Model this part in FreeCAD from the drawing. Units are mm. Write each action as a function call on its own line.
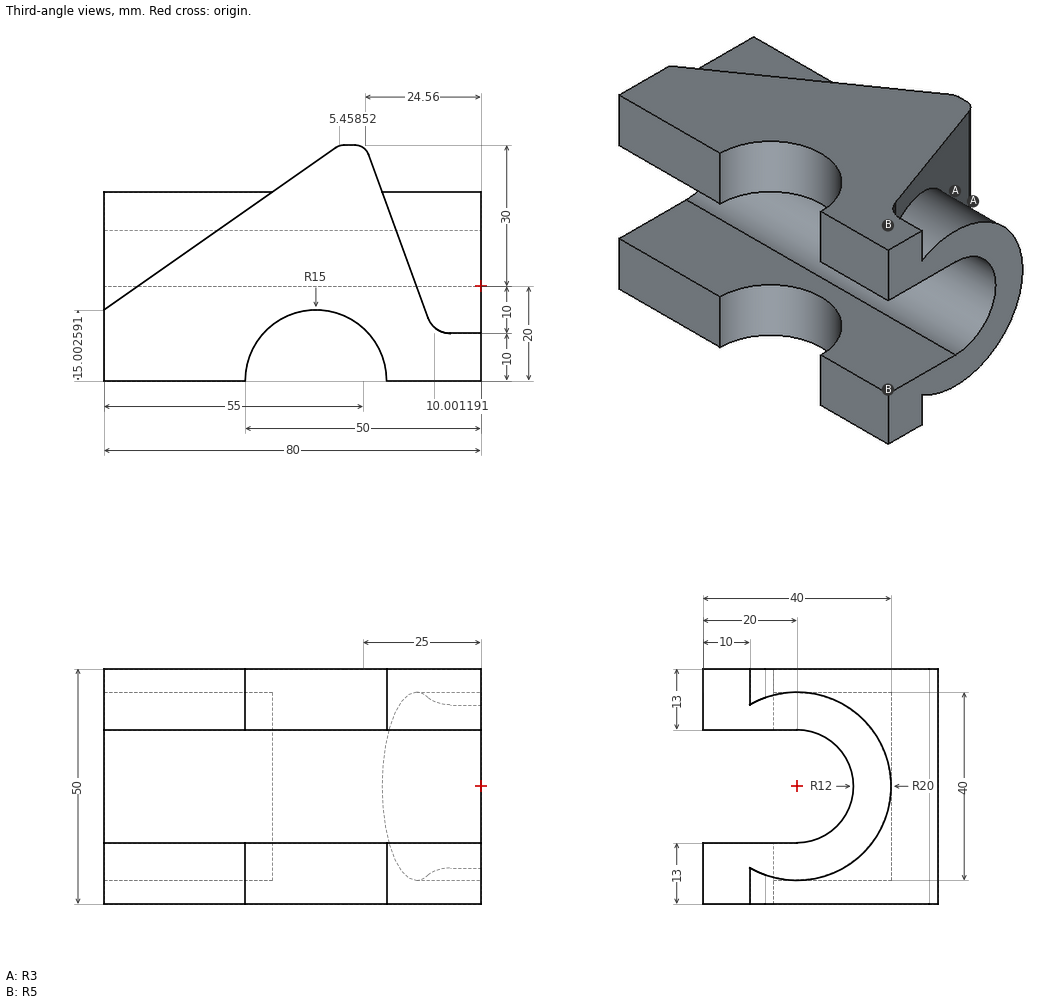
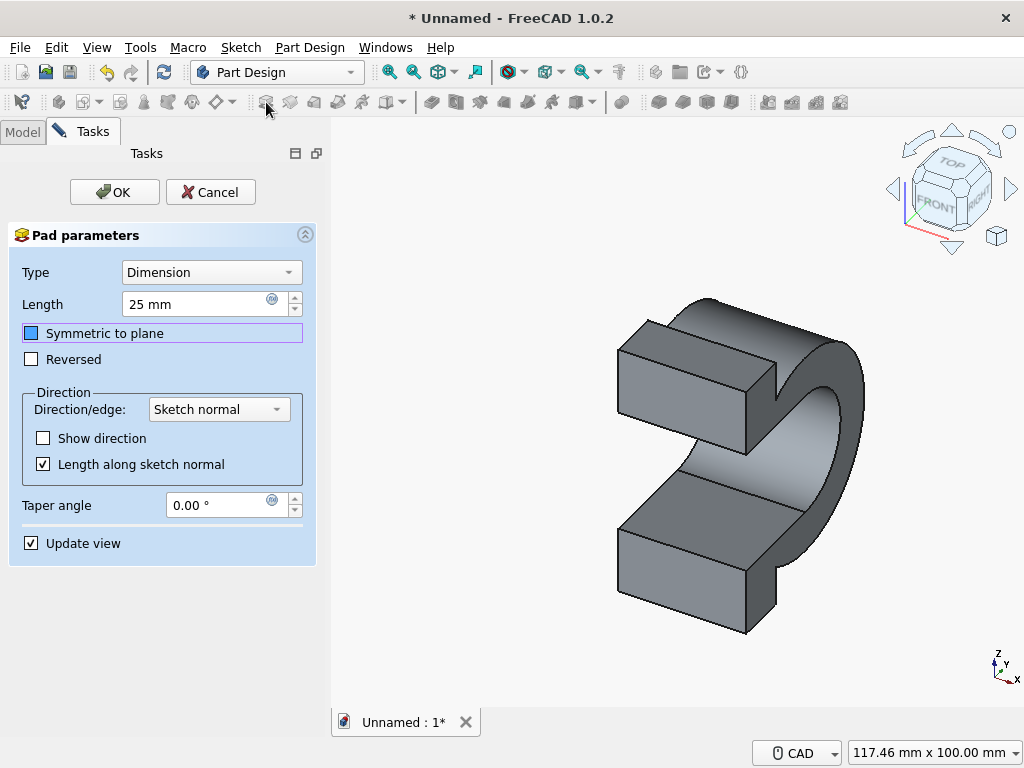
click(30, 359)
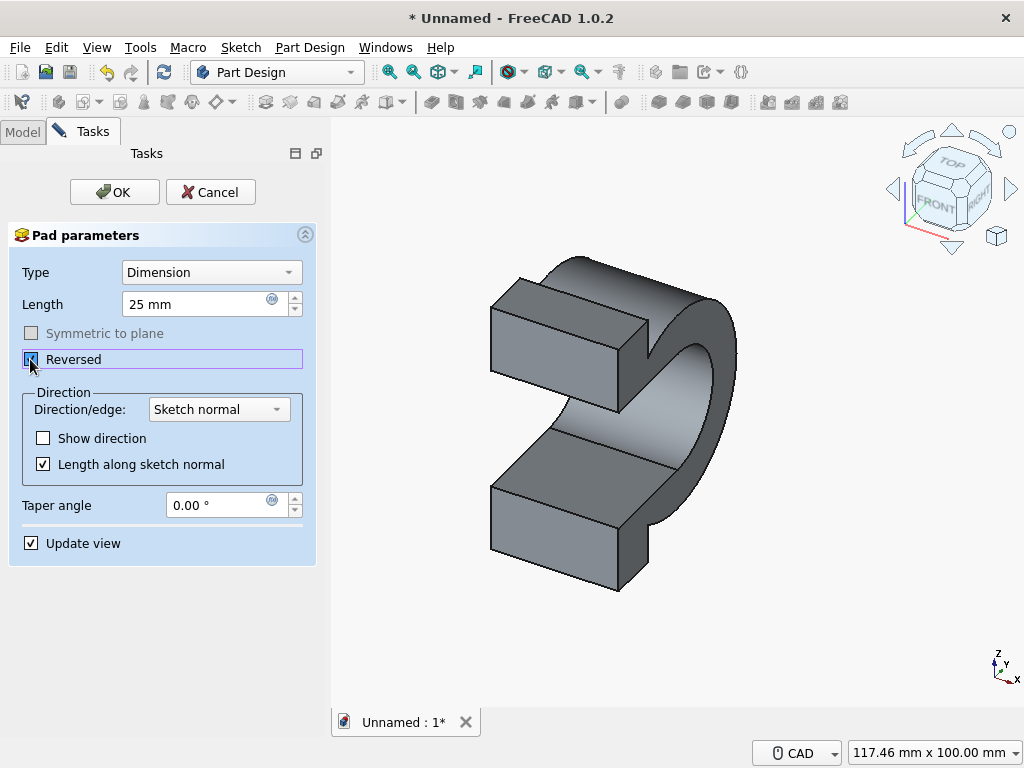
click(115, 192)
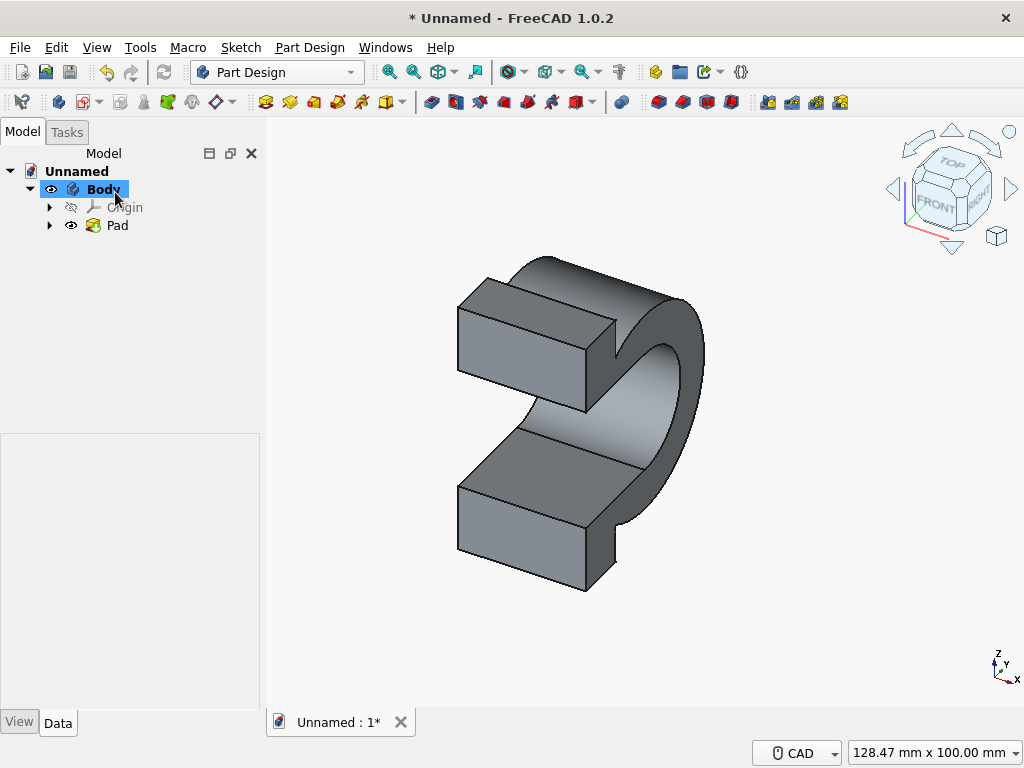
key(6)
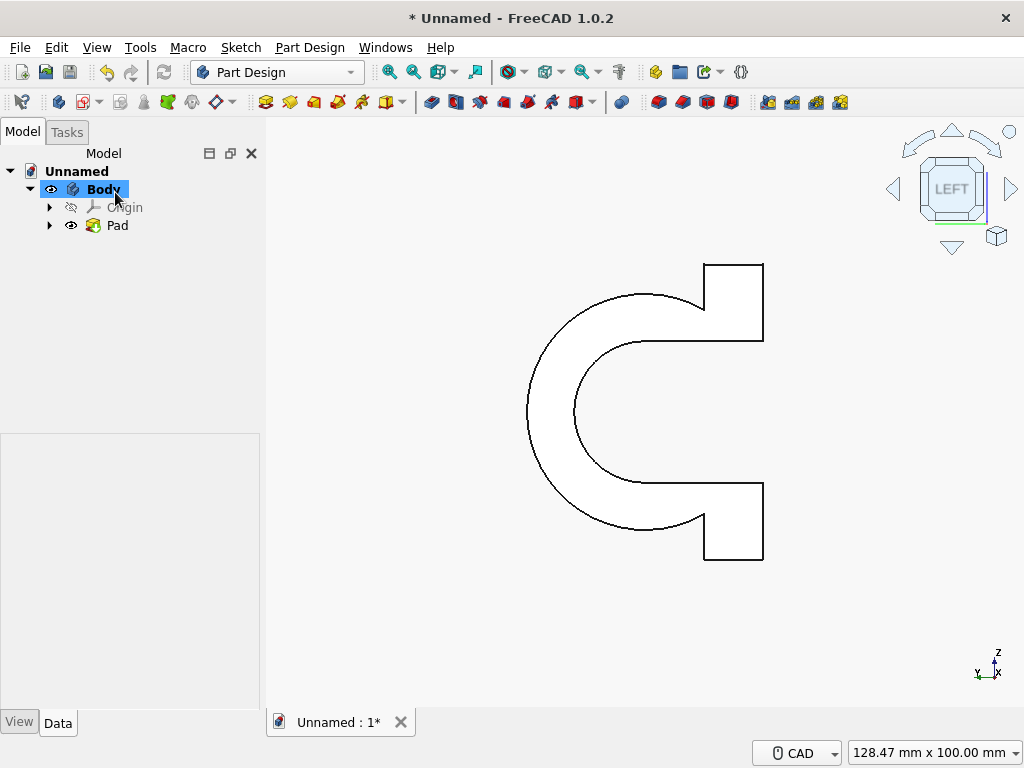
click(611, 327)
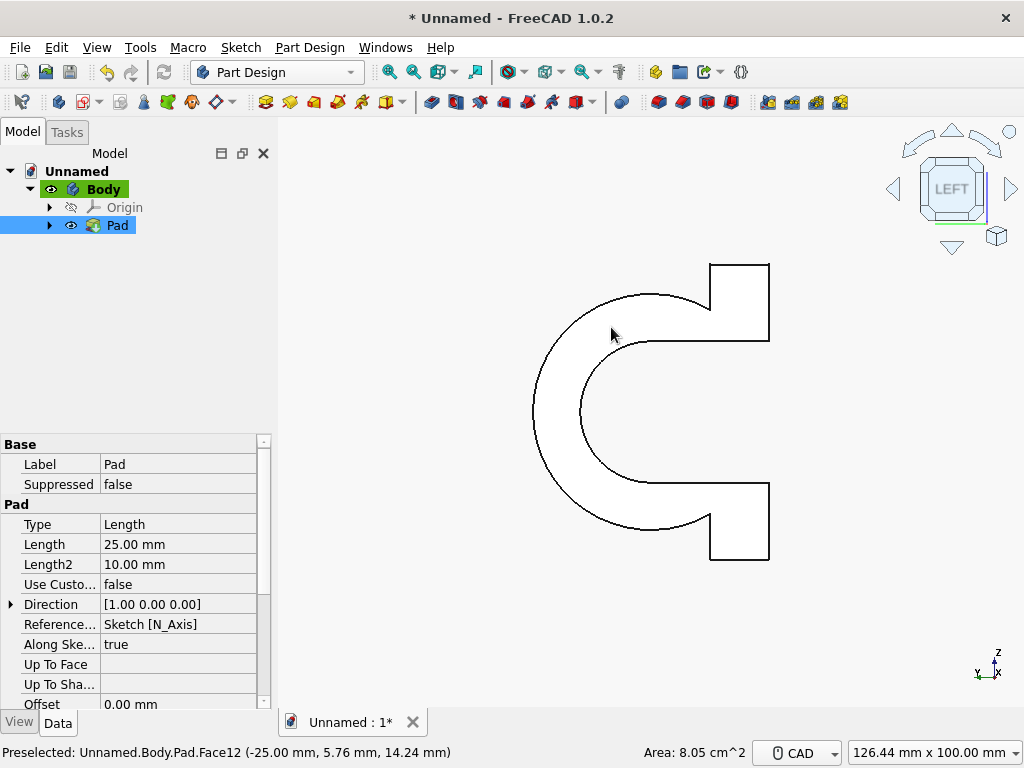
click(84, 102)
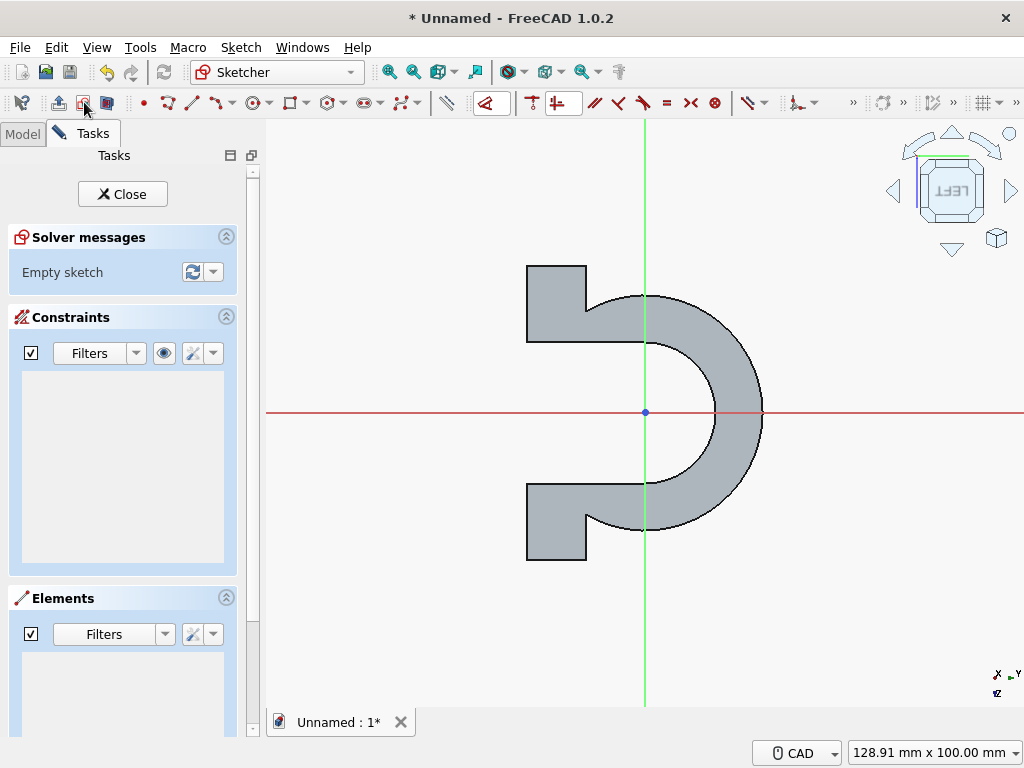
scroll(784, 413, up, 2)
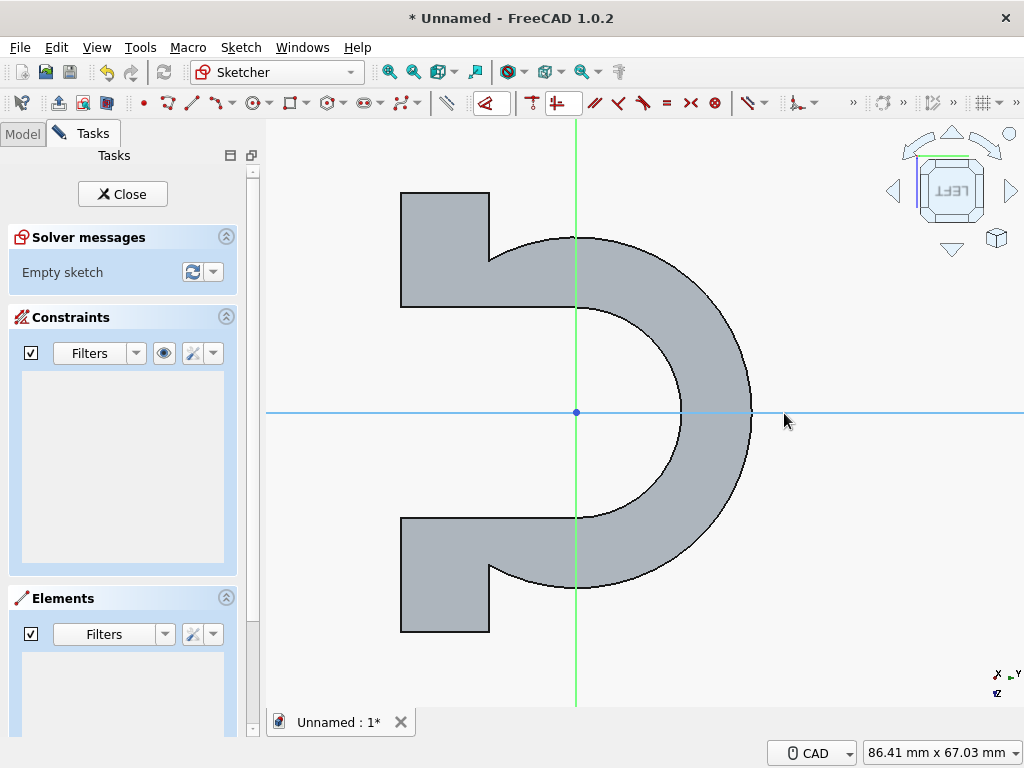
click(308, 104)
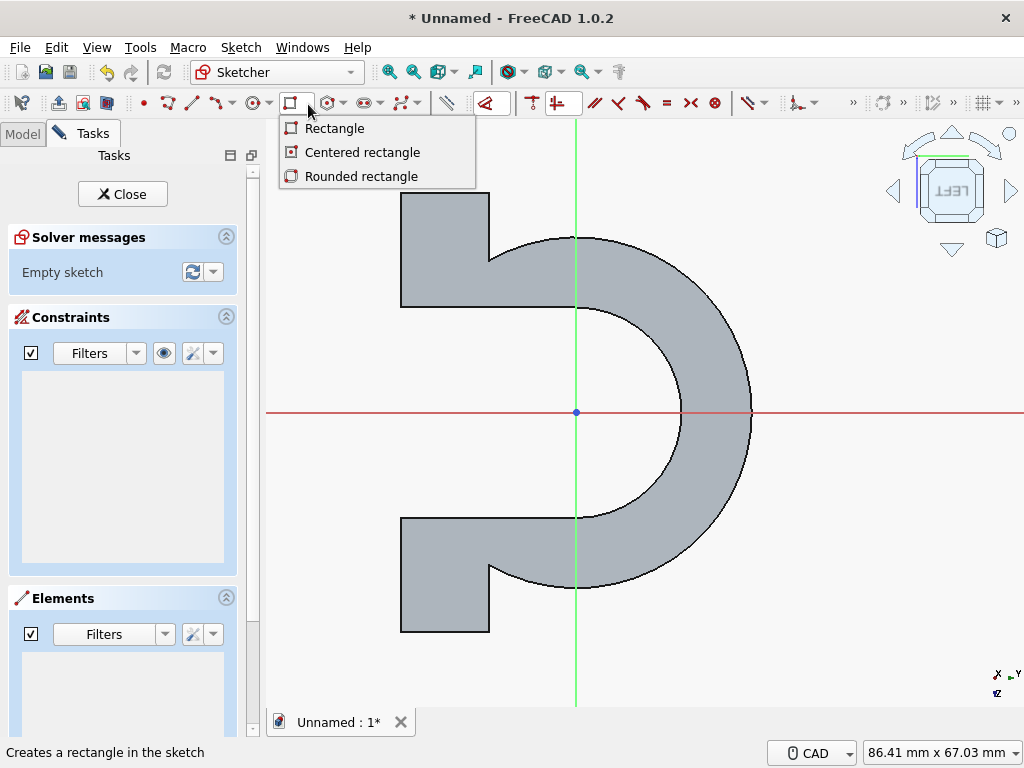
click(378, 152)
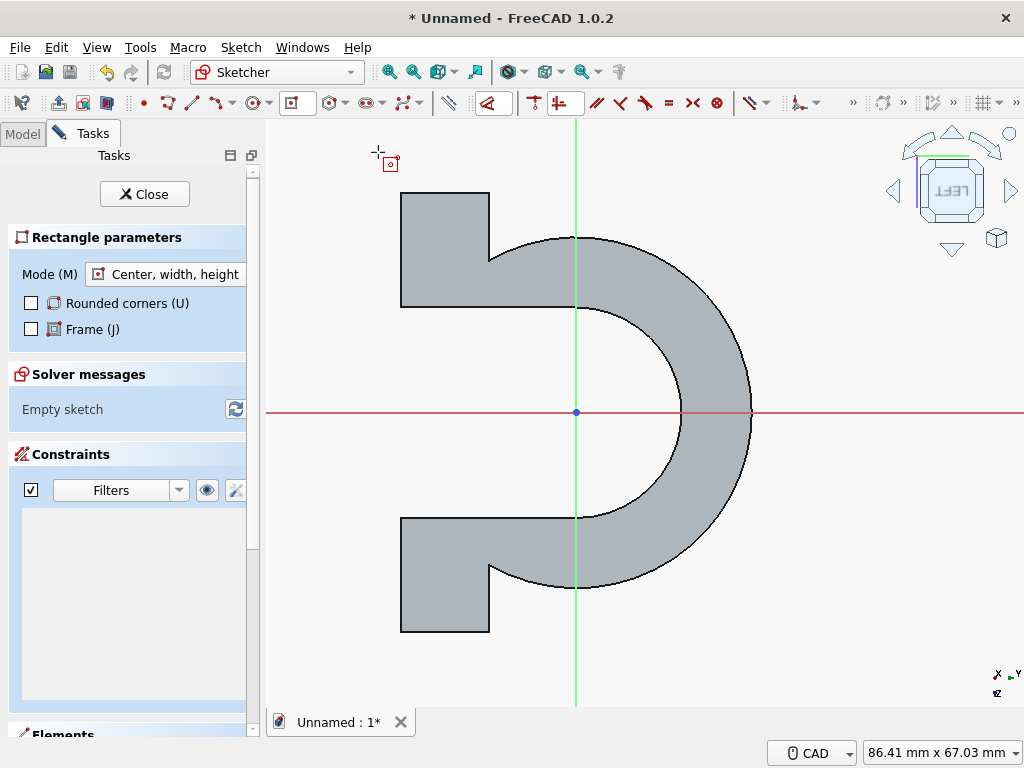
click(576, 413)
move(752, 237)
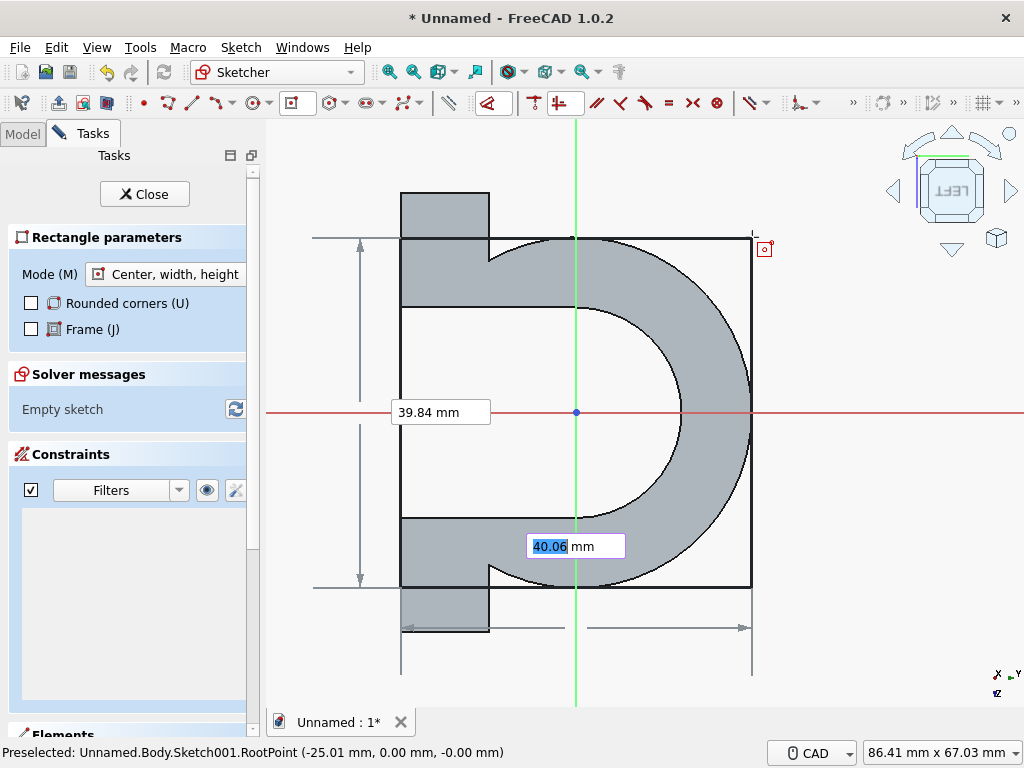
text(40)
key(Tab)
text(40)
key(Return)
key(Escape)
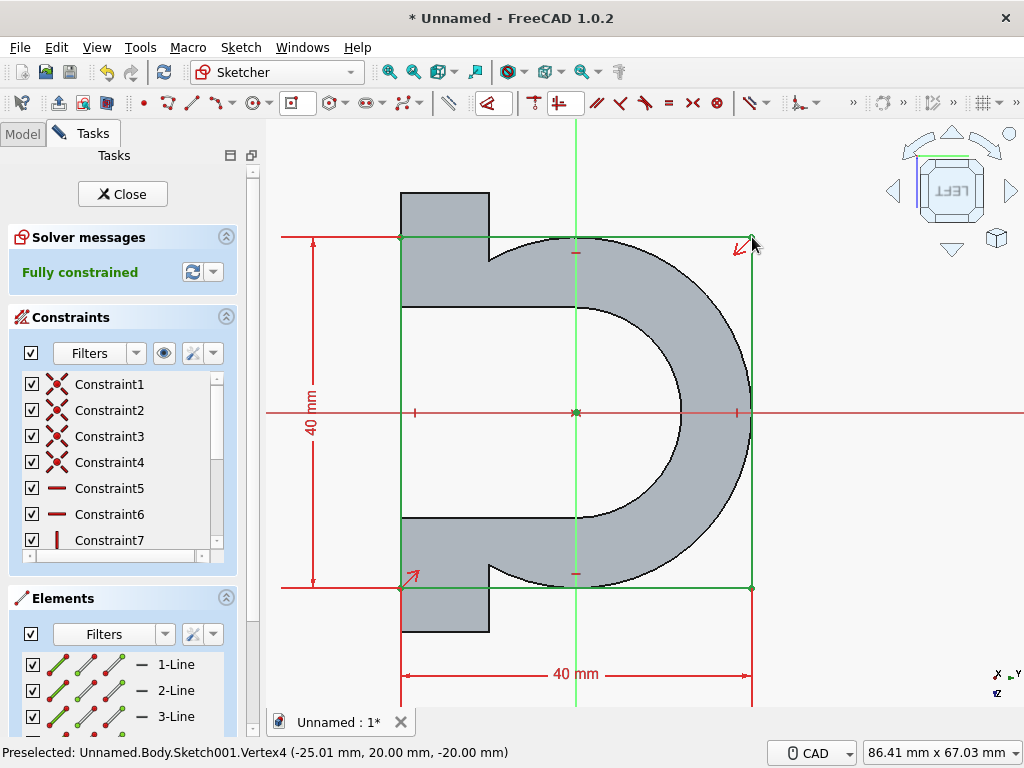
click(123, 194)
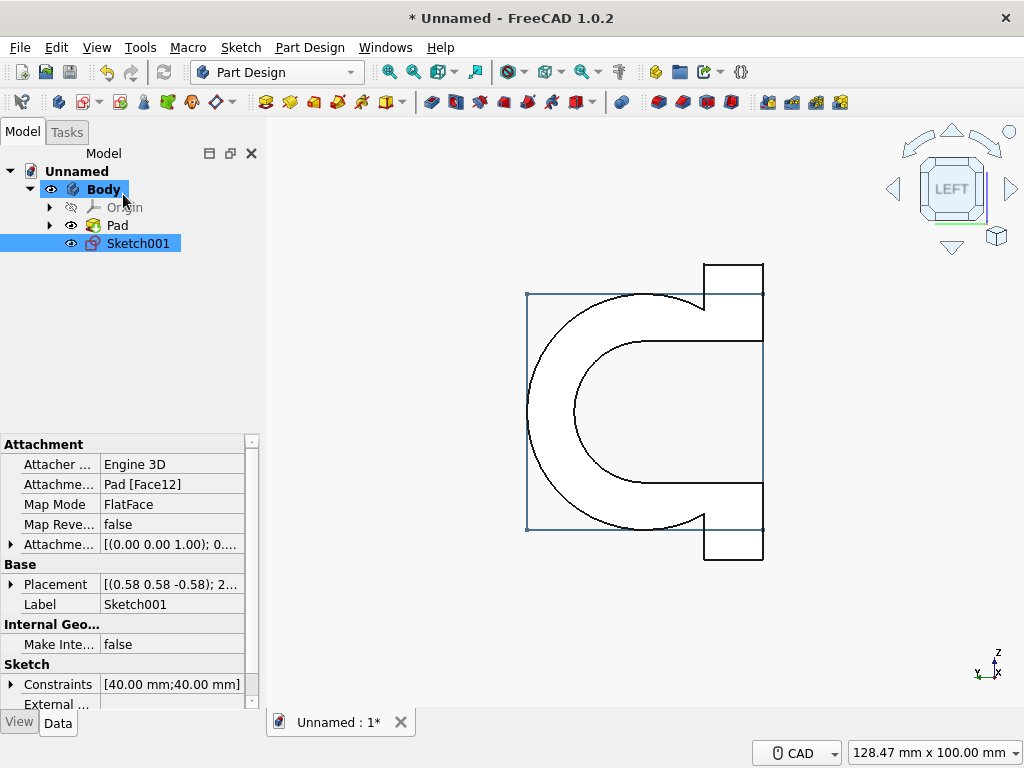
click(266, 102)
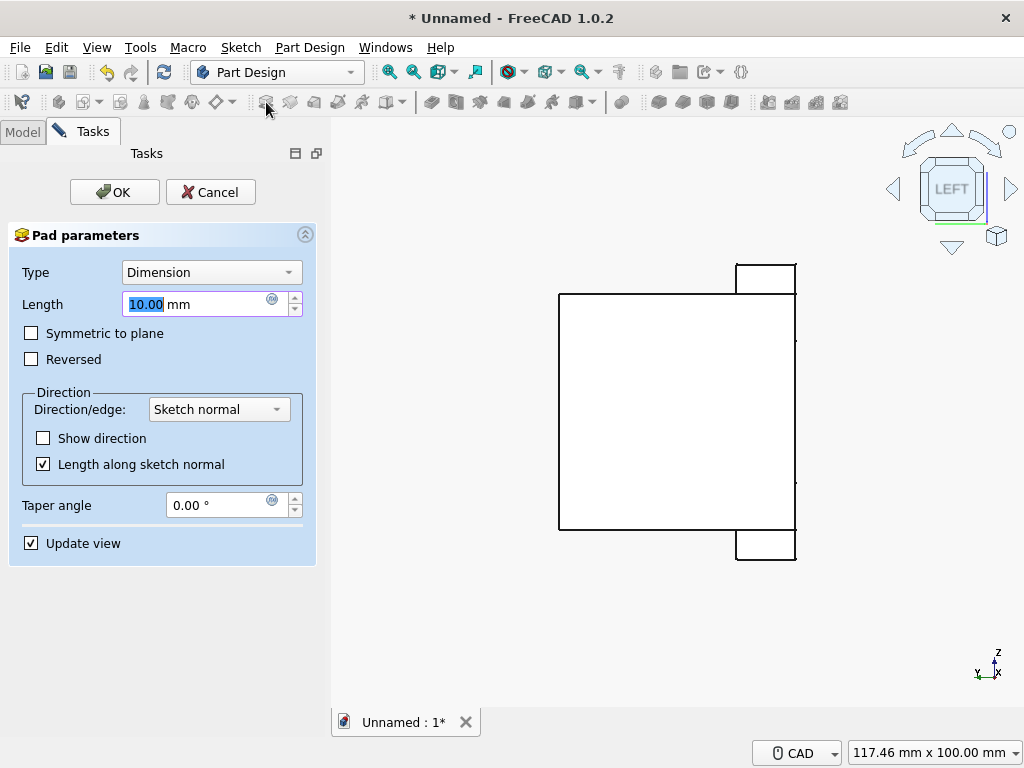
text(55)
key(Tab)